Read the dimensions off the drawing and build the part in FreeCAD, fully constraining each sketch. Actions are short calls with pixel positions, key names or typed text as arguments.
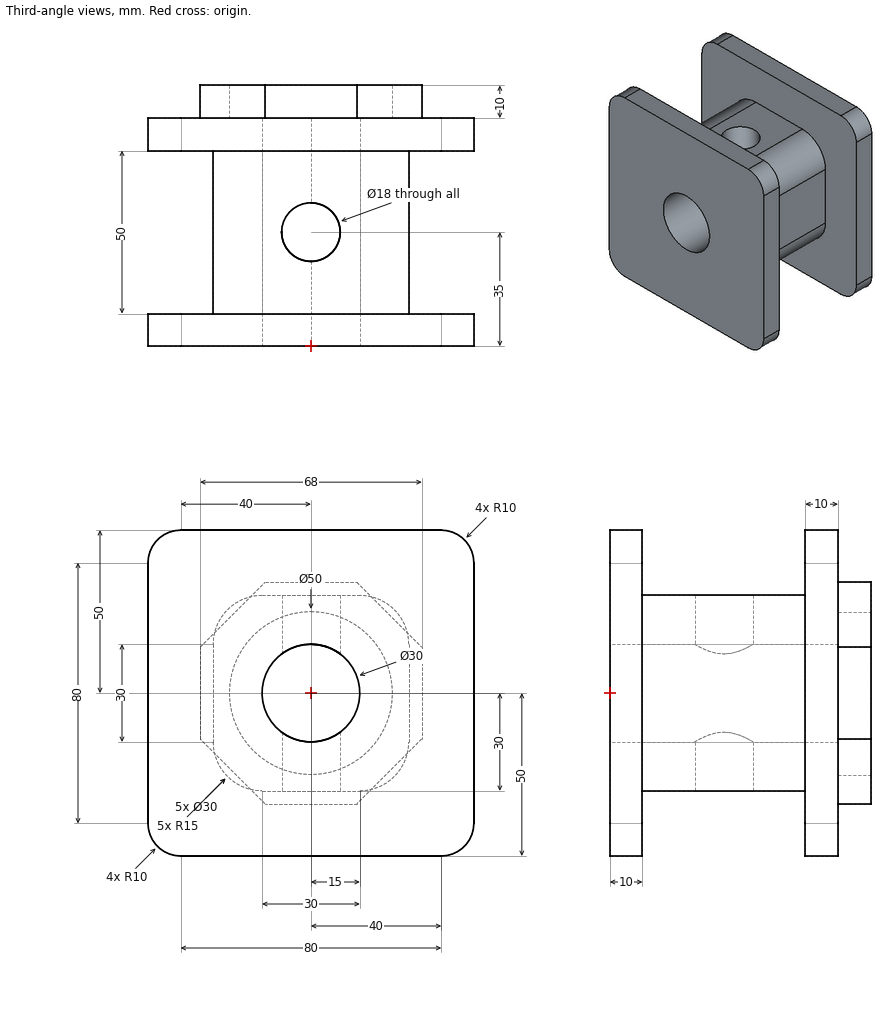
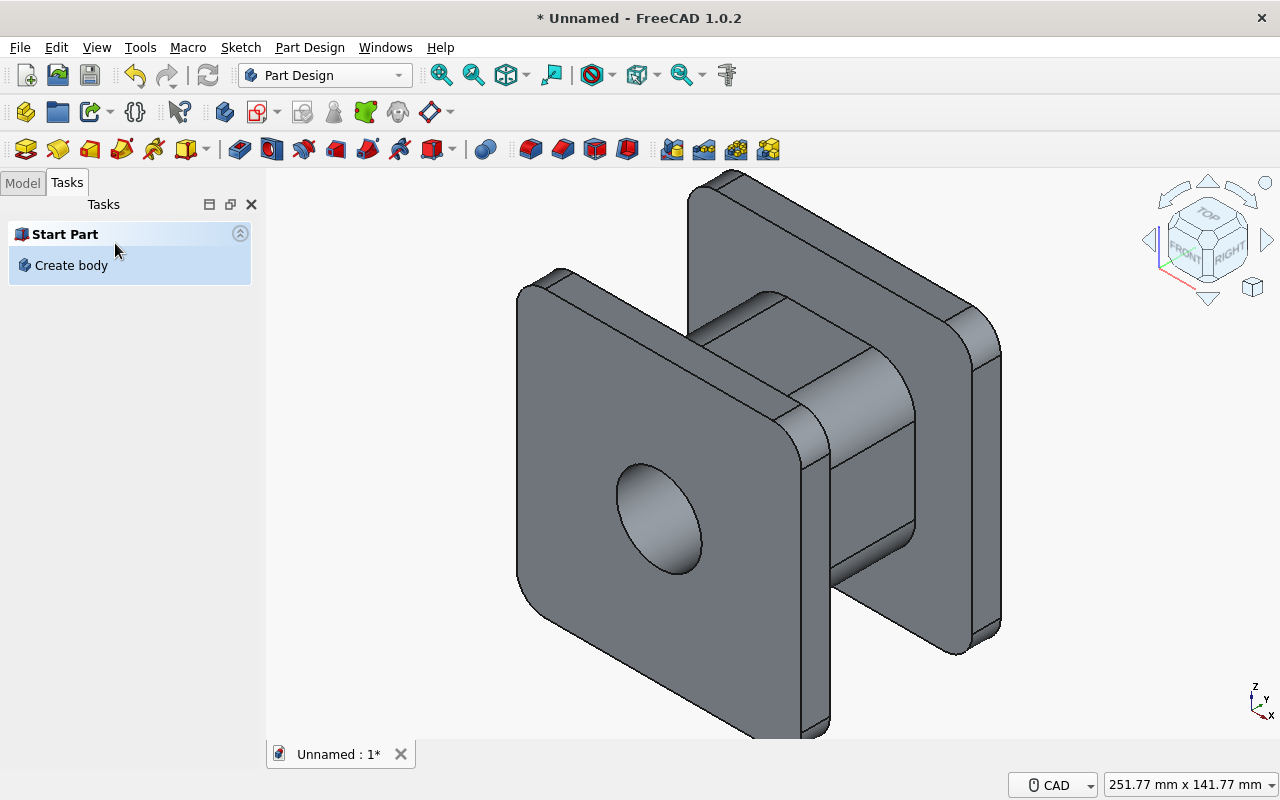
click(442, 76)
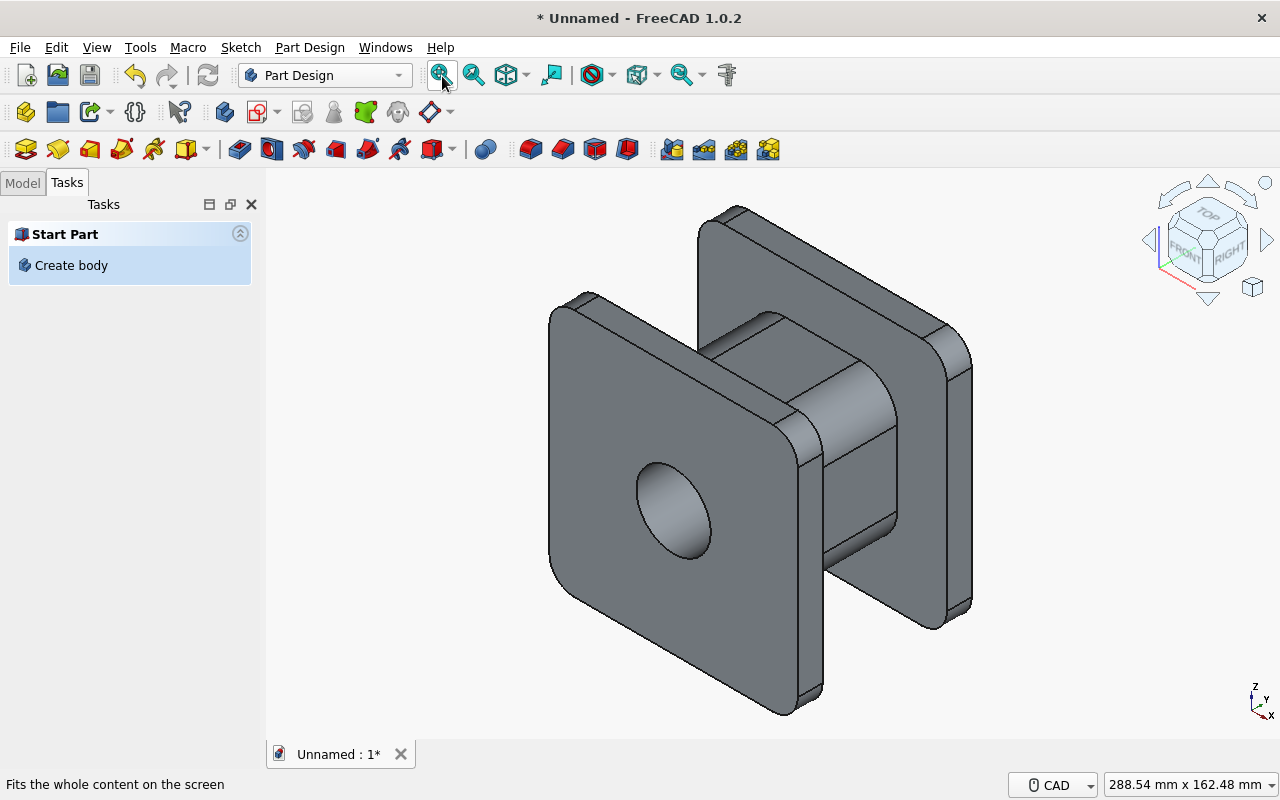
click(778, 363)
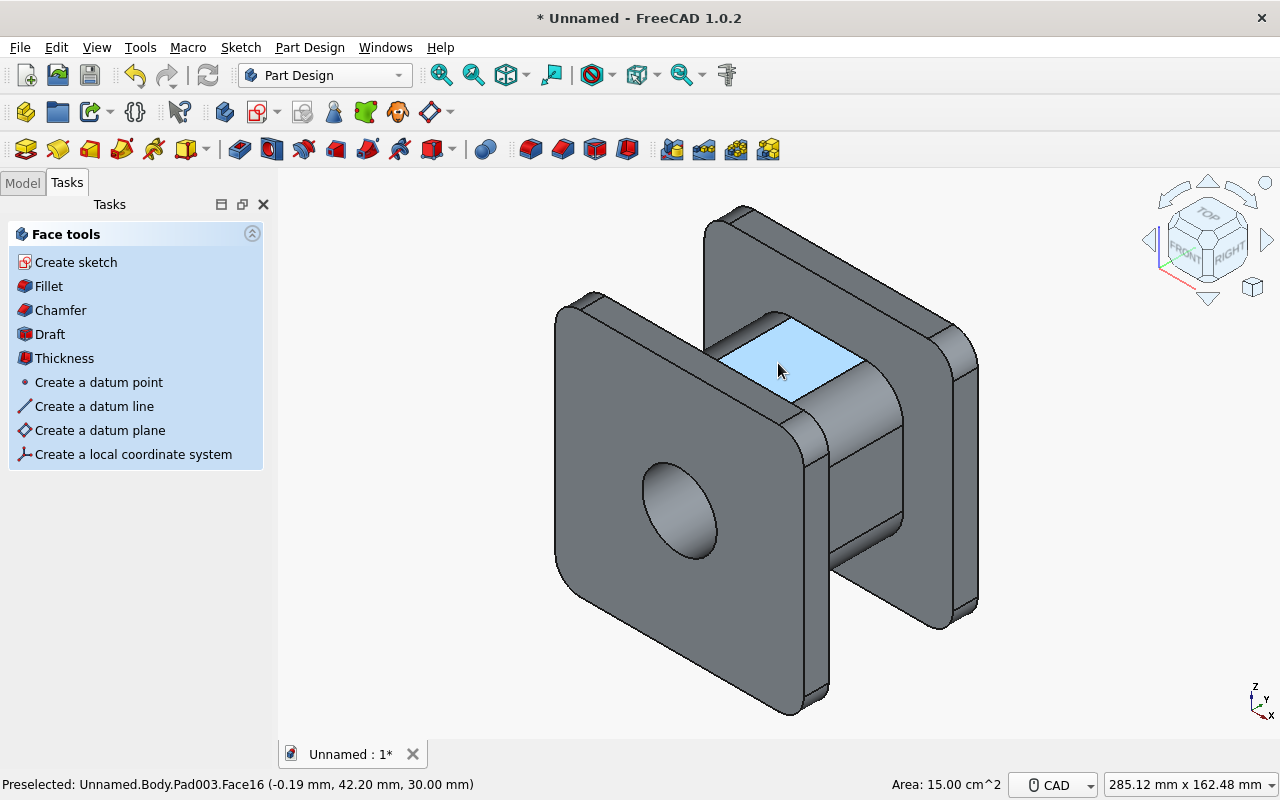
click(258, 112)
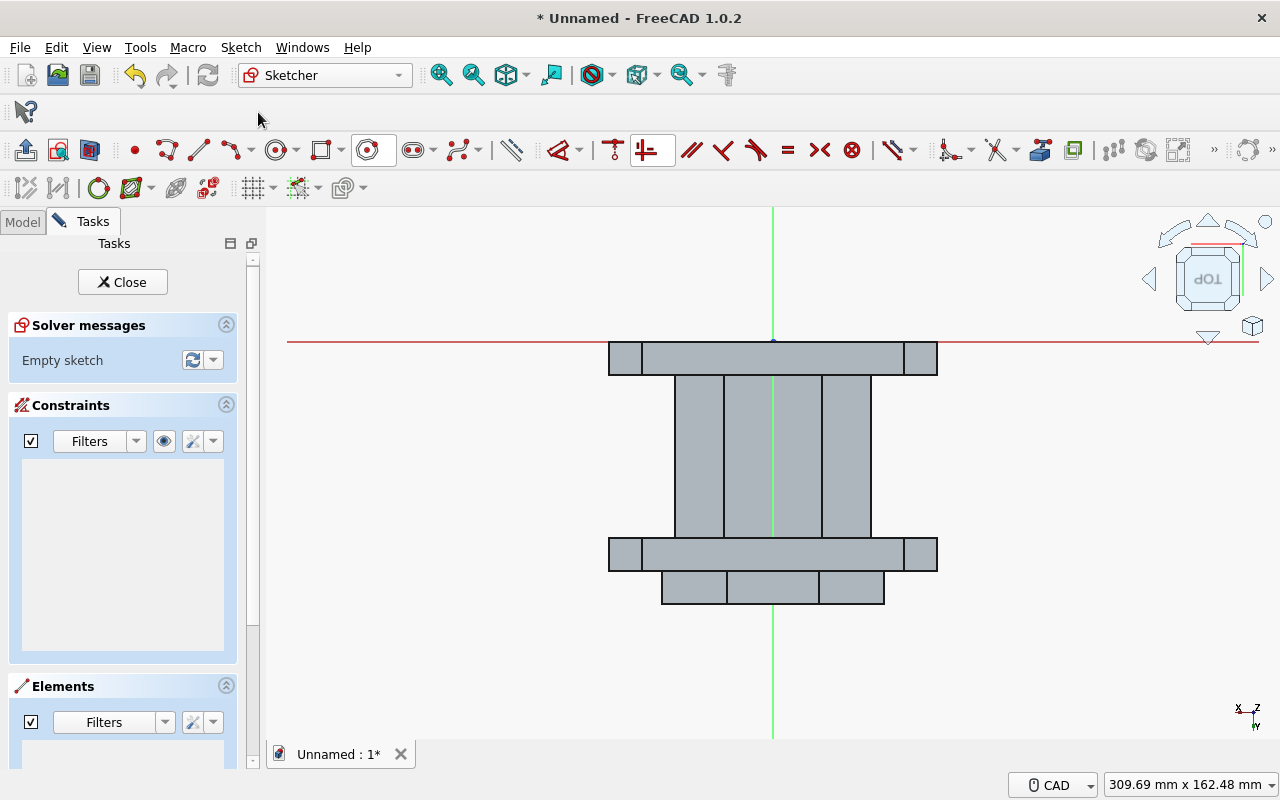
click(90, 150)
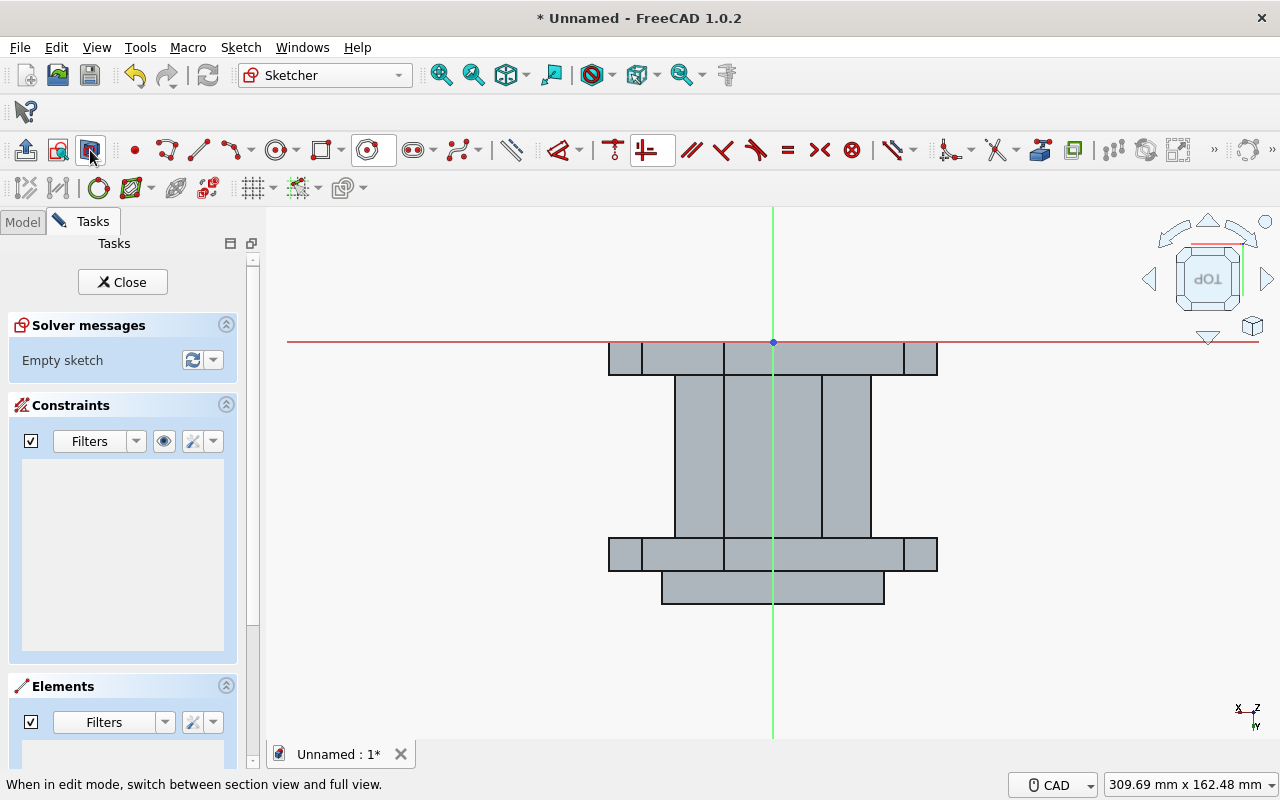
scroll(829, 366, up, 4)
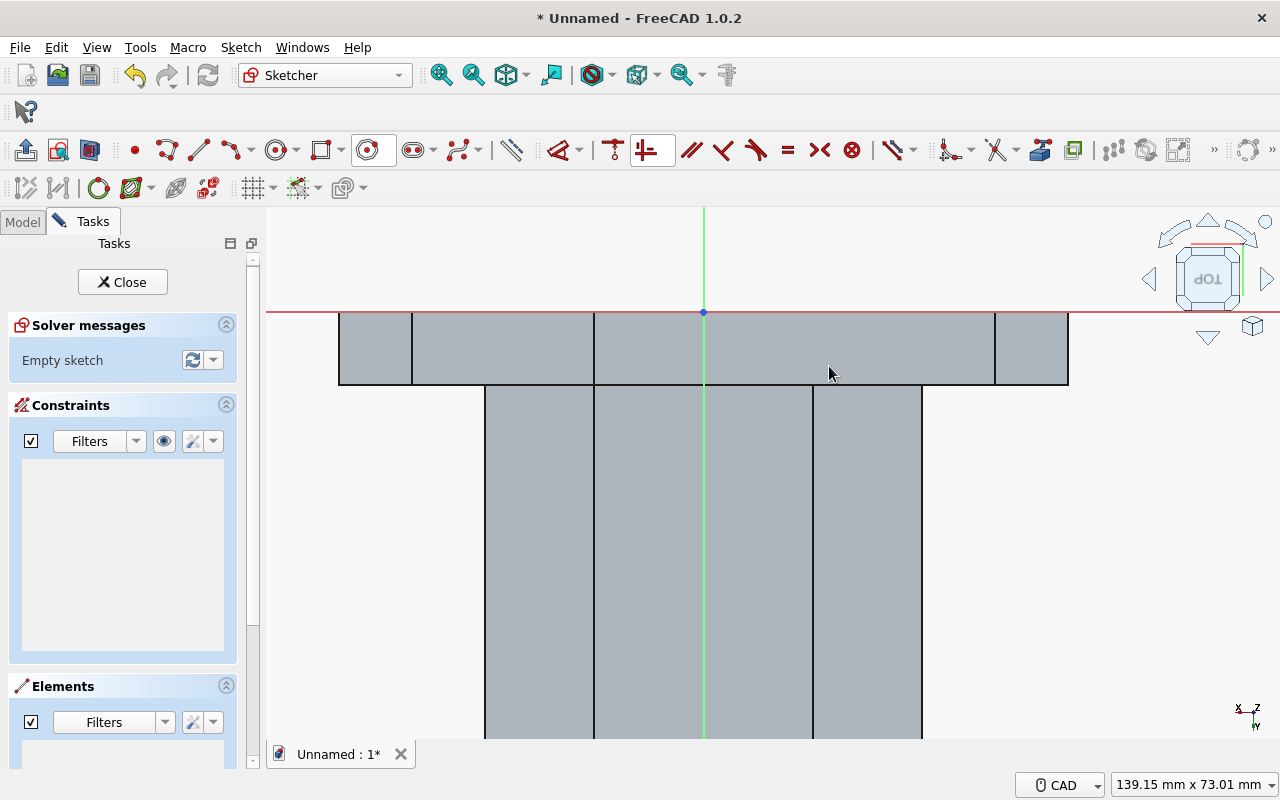
click(276, 150)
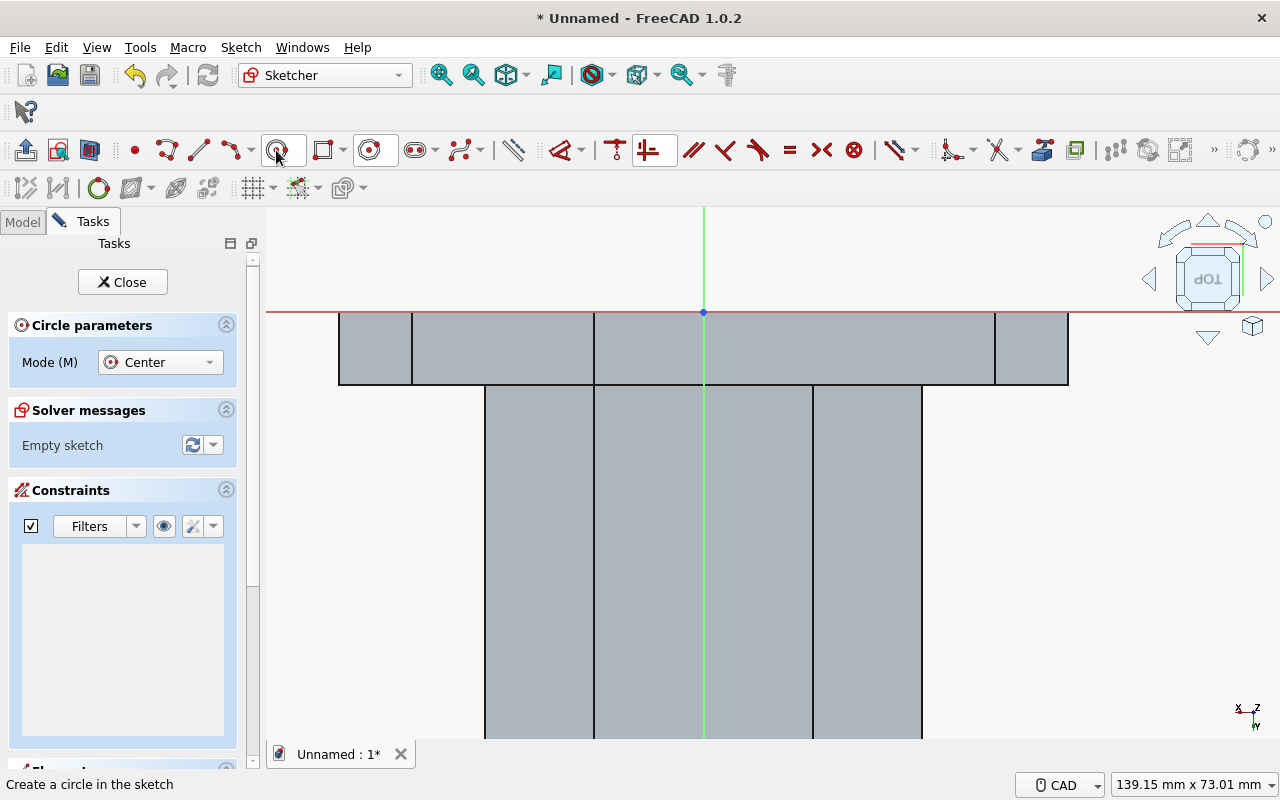
click(704, 567)
move(750, 521)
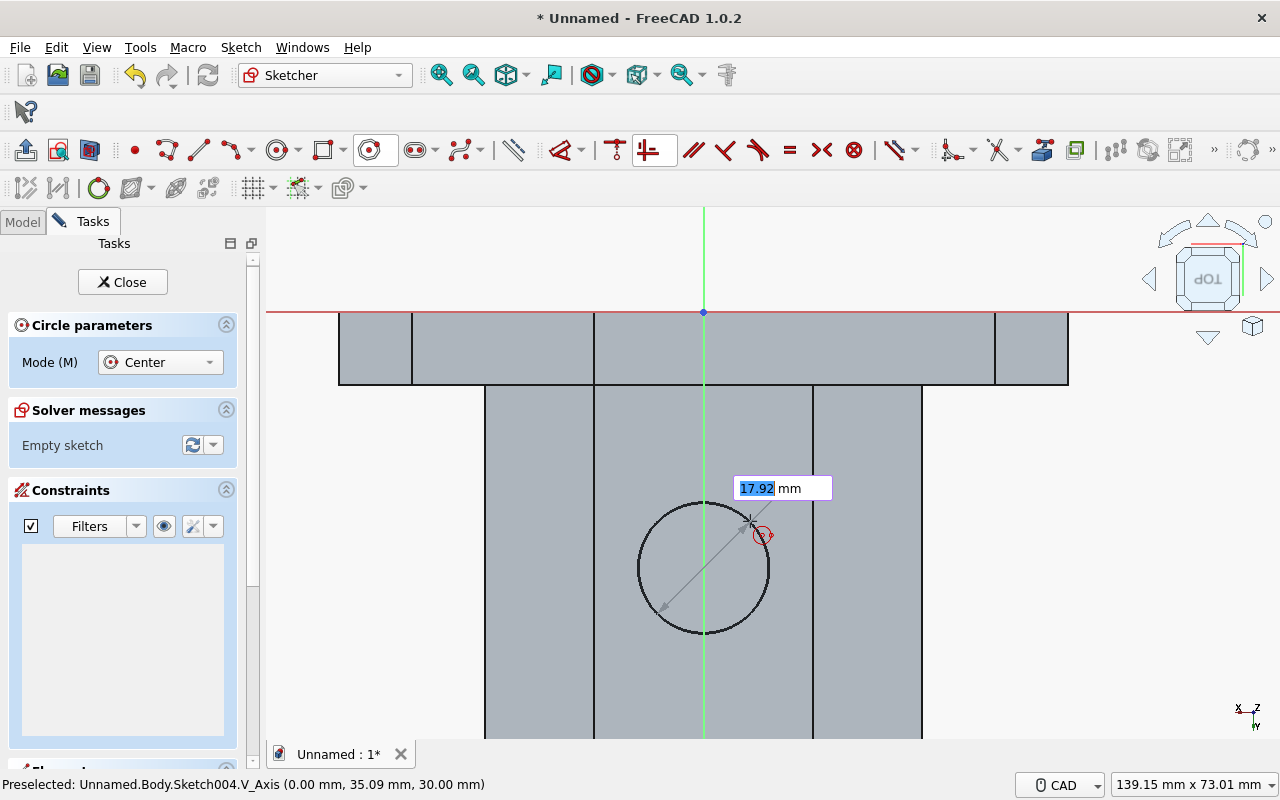
text(18)
key(Return)
key(Escape)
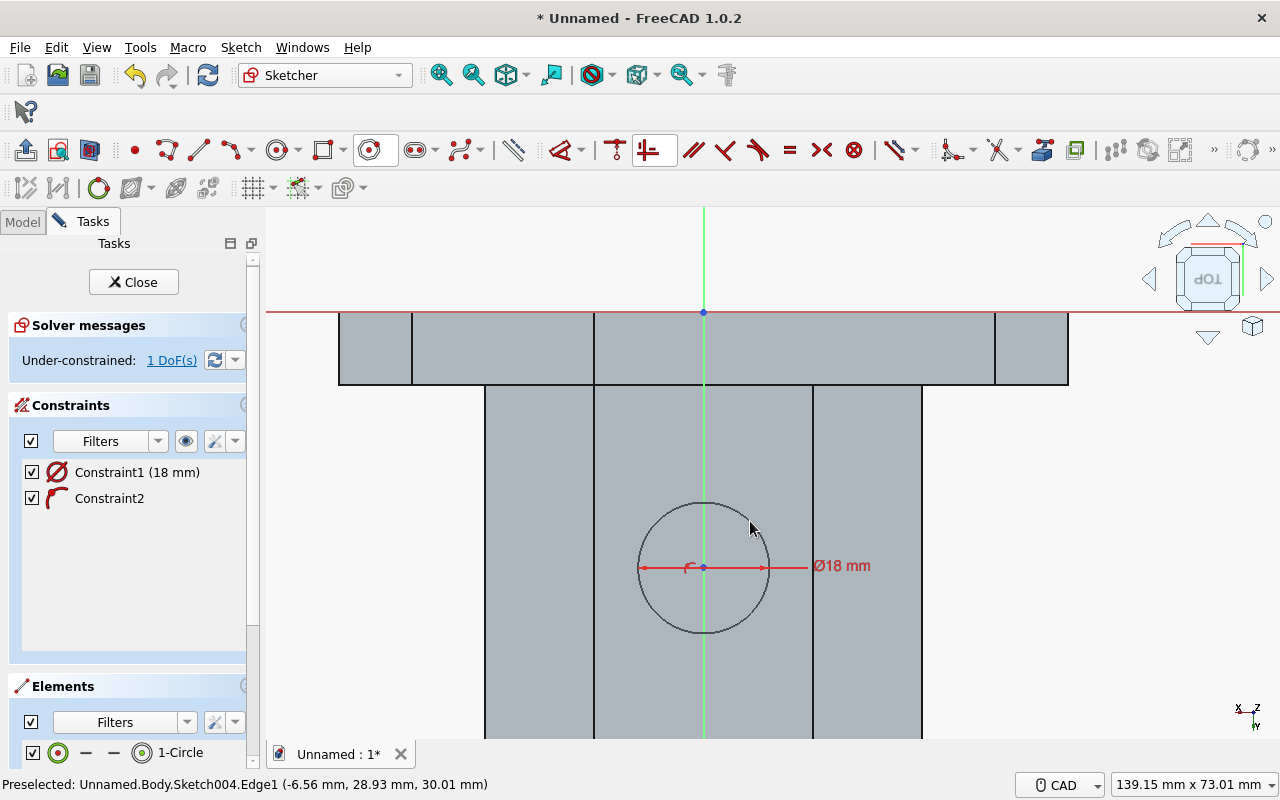
click(560, 150)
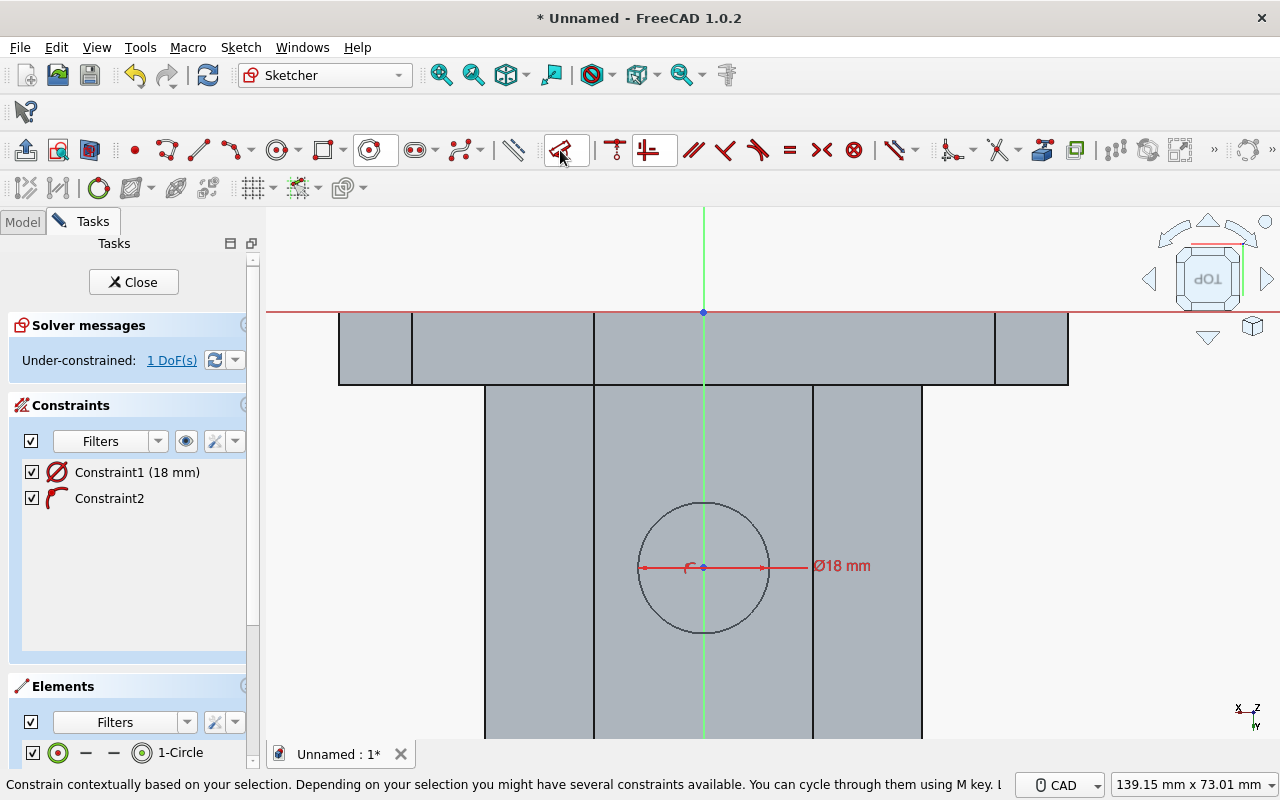
click(704, 568)
click(738, 440)